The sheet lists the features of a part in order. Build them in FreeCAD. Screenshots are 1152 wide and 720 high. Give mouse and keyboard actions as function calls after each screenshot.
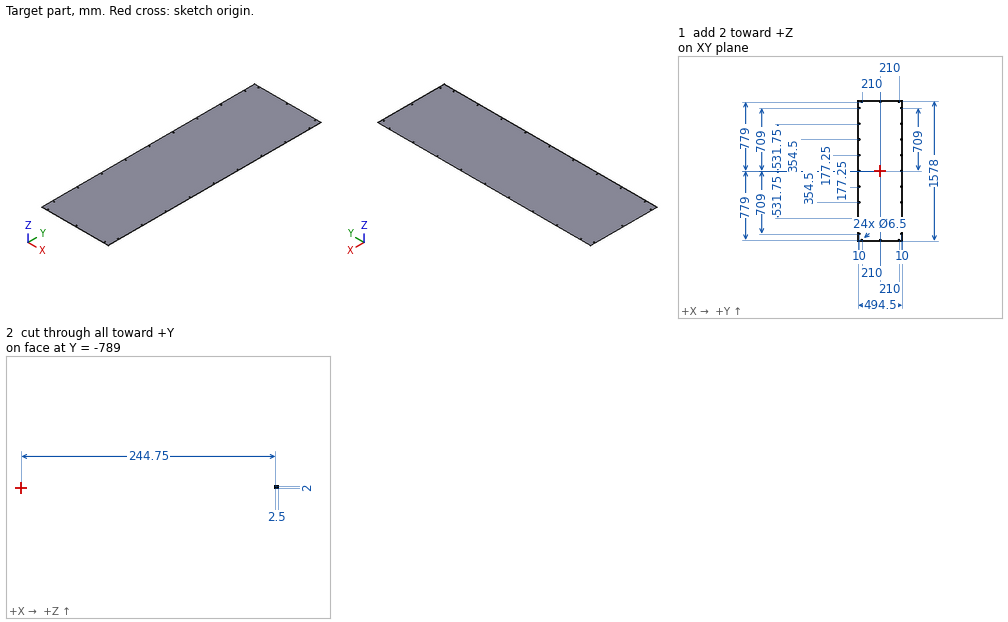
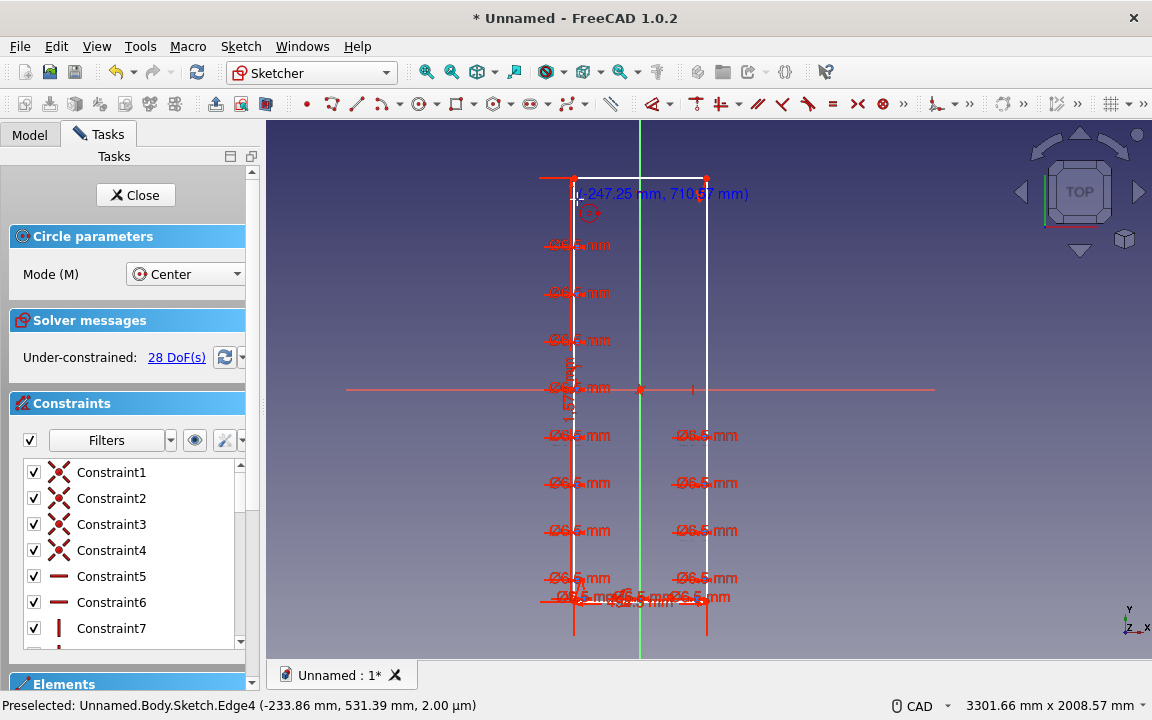
scroll(577, 200, up, 9)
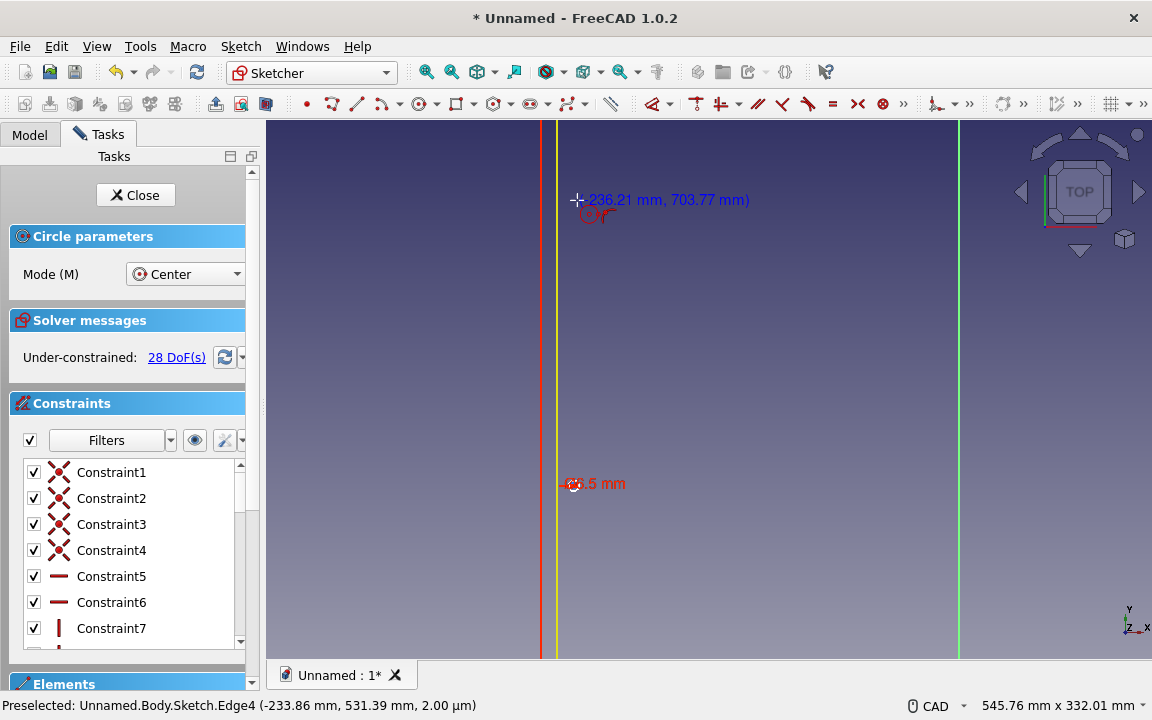
click(574, 197)
move(577, 193)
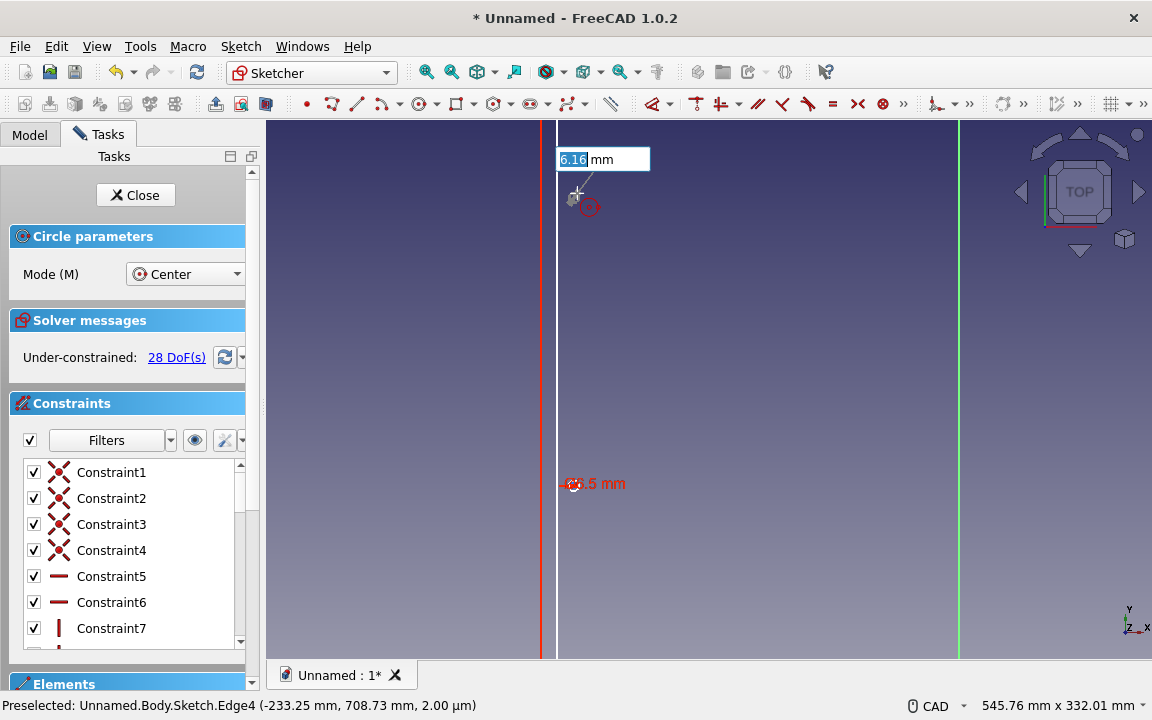
text(6.5)
key(Return)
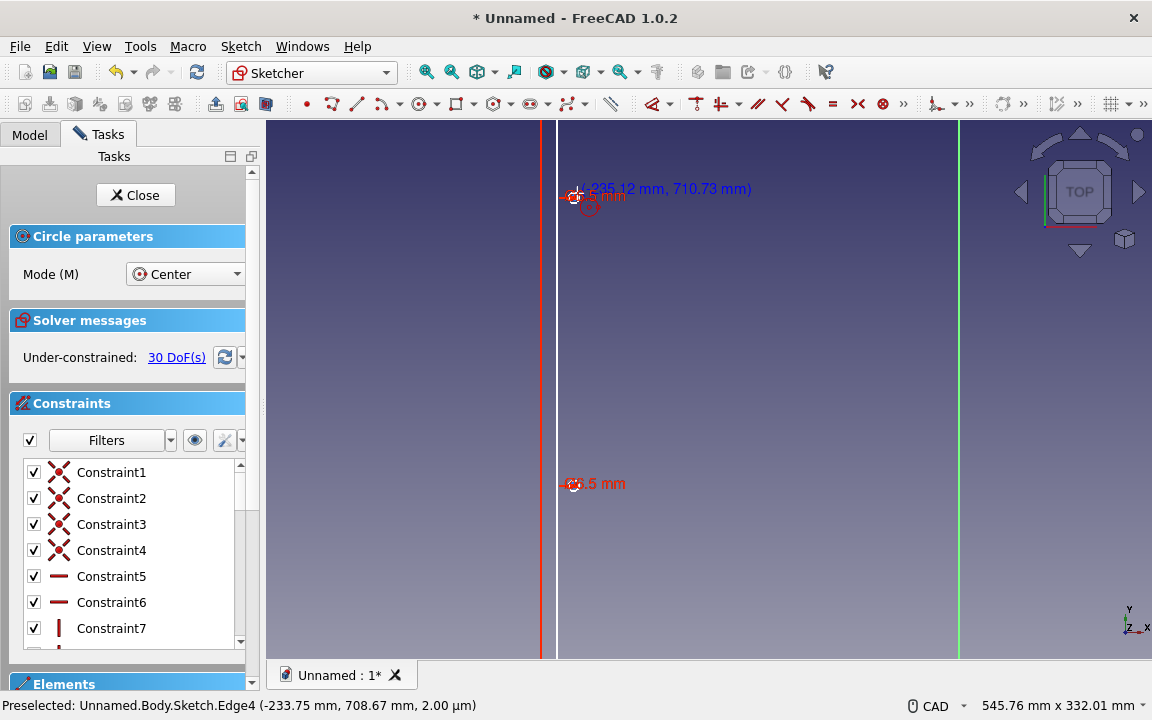
scroll(591, 240, down, 10)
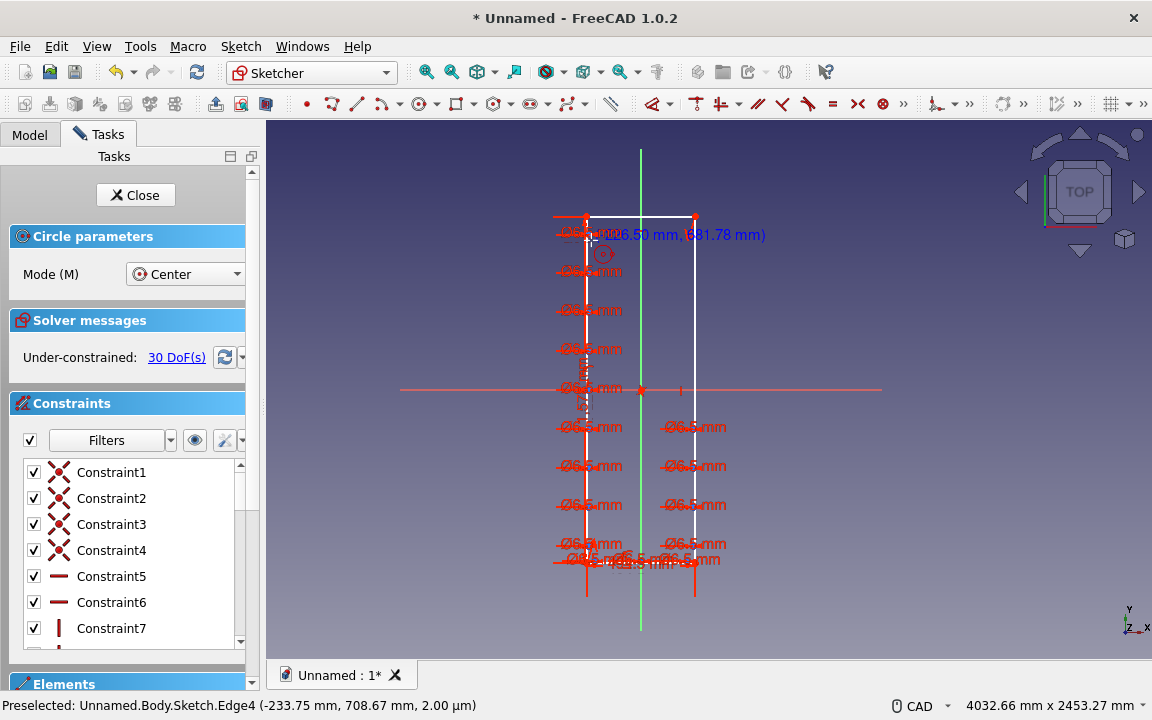
scroll(595, 219, up, 18)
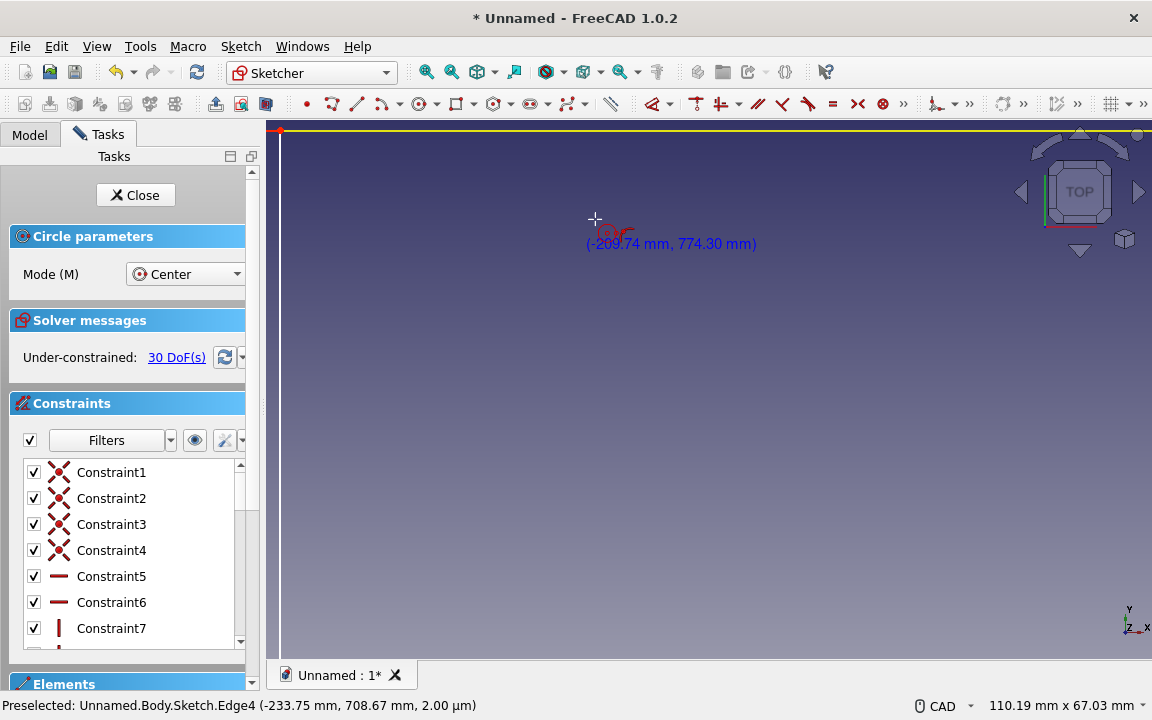
scroll(584, 179, down, 17)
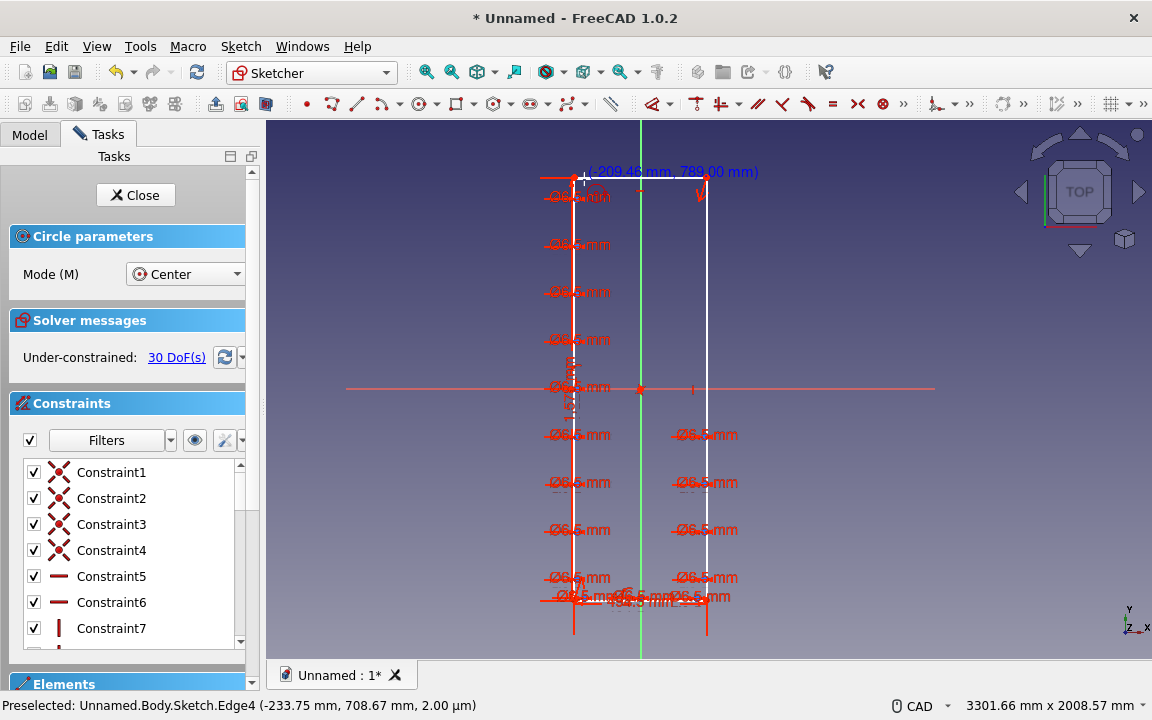
scroll(584, 180, up, 9)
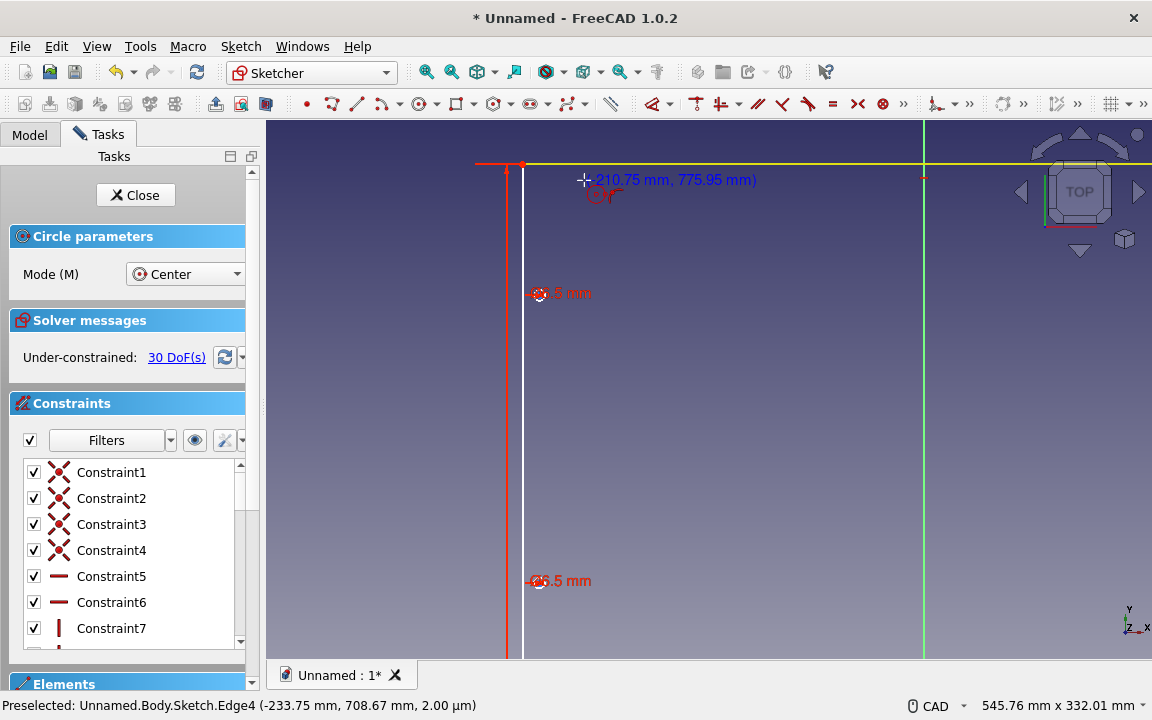
click(583, 181)
move(587, 184)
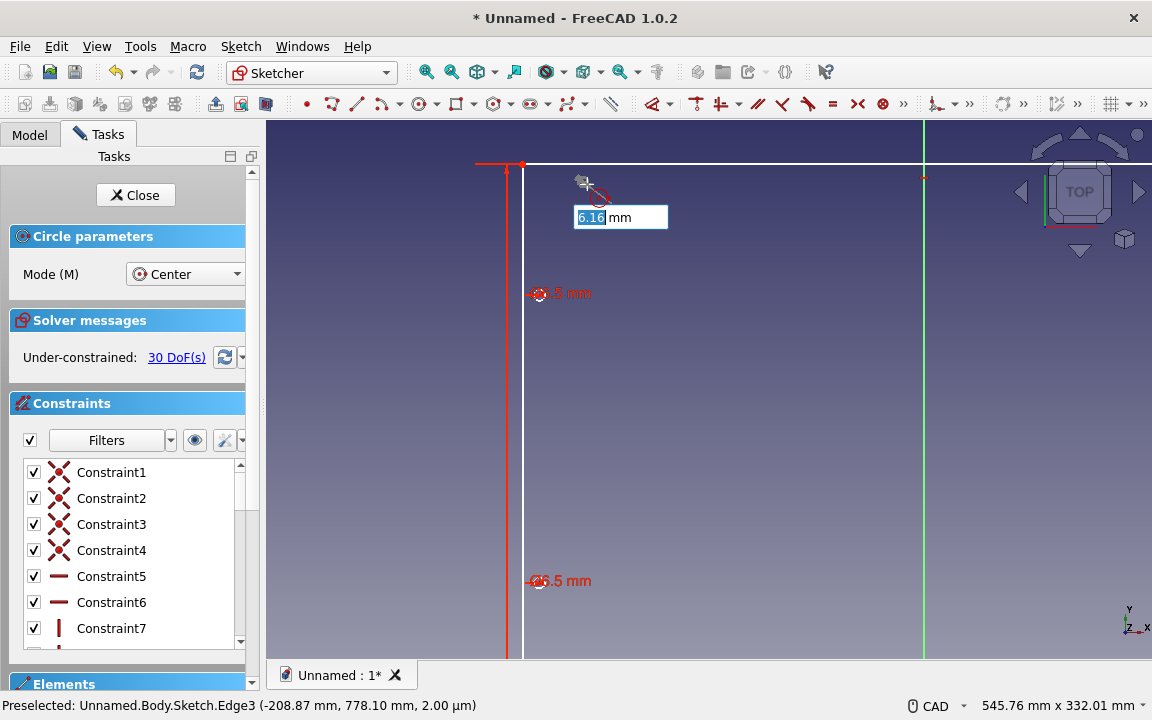
text(6.5)
key(Return)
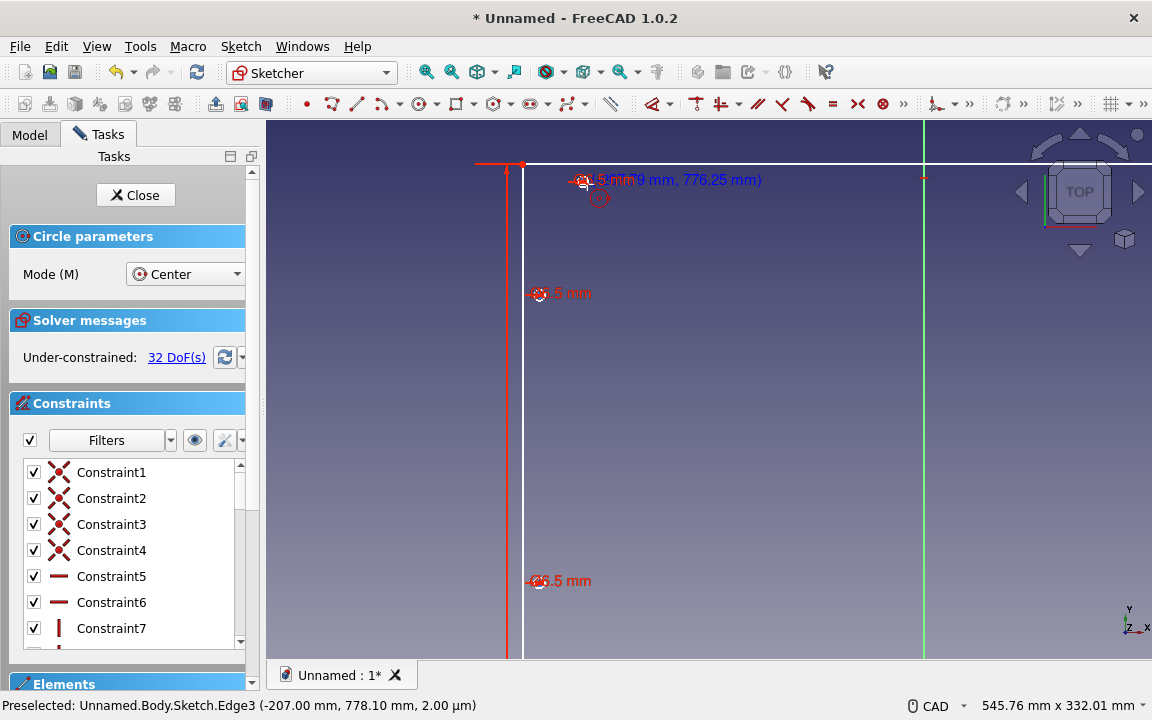
scroll(596, 224, down, 10)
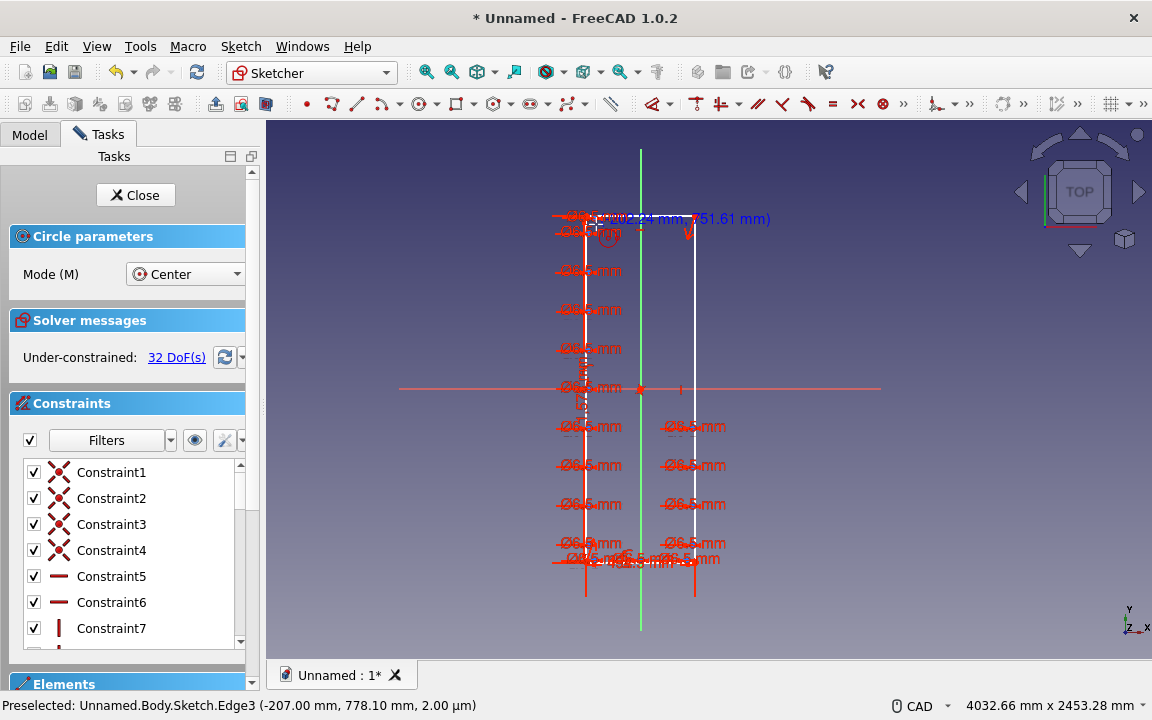
scroll(693, 389, up, 18)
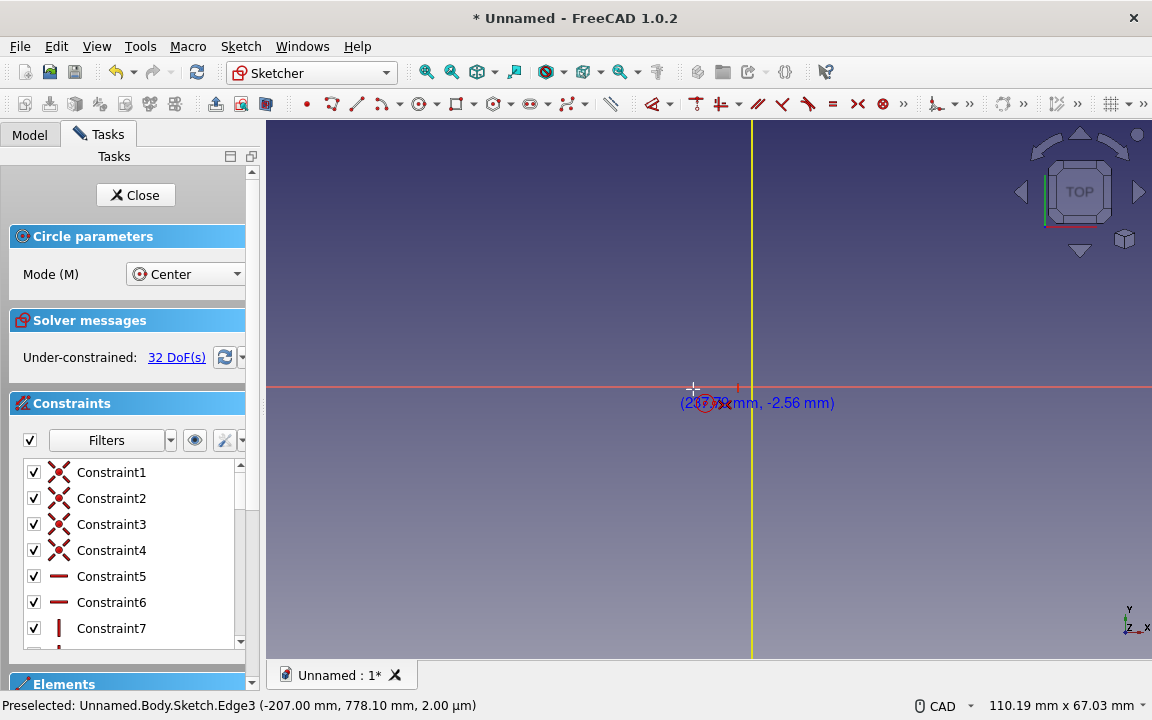
scroll(705, 390, down, 17)